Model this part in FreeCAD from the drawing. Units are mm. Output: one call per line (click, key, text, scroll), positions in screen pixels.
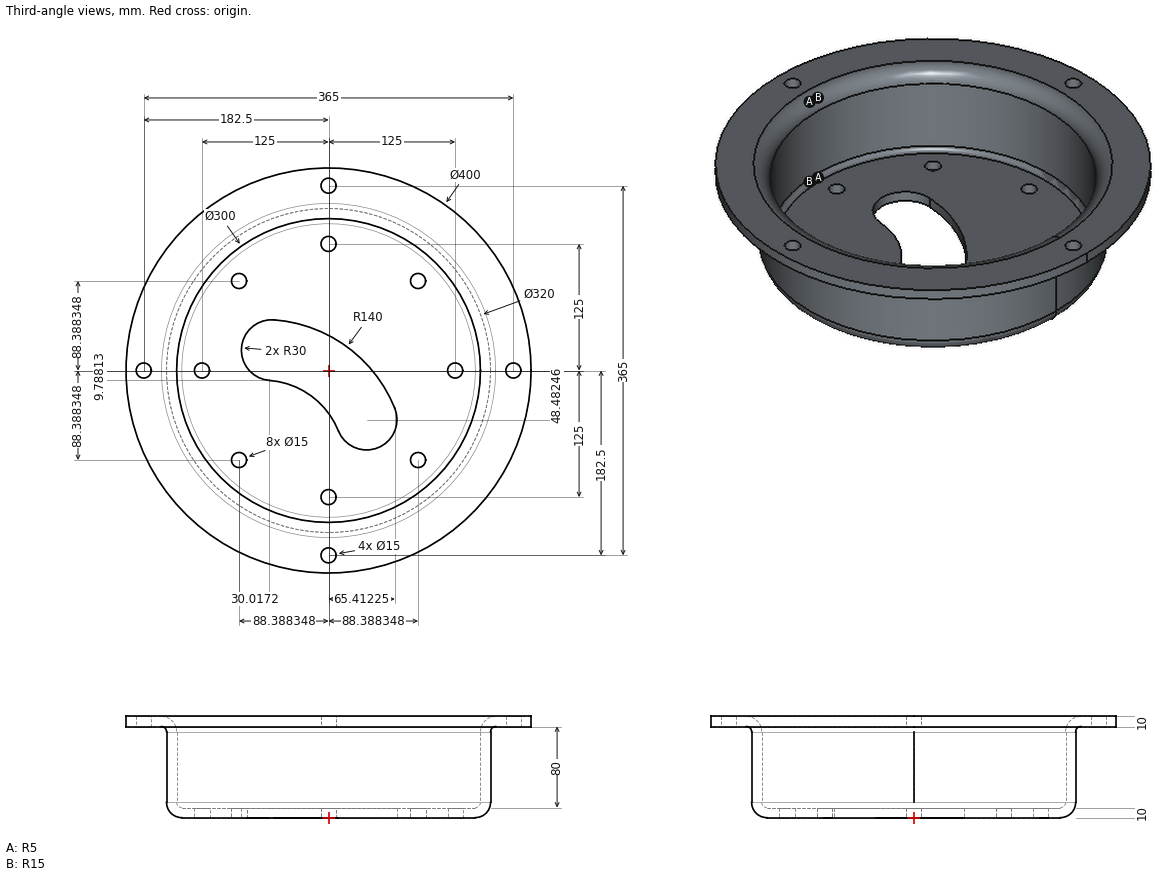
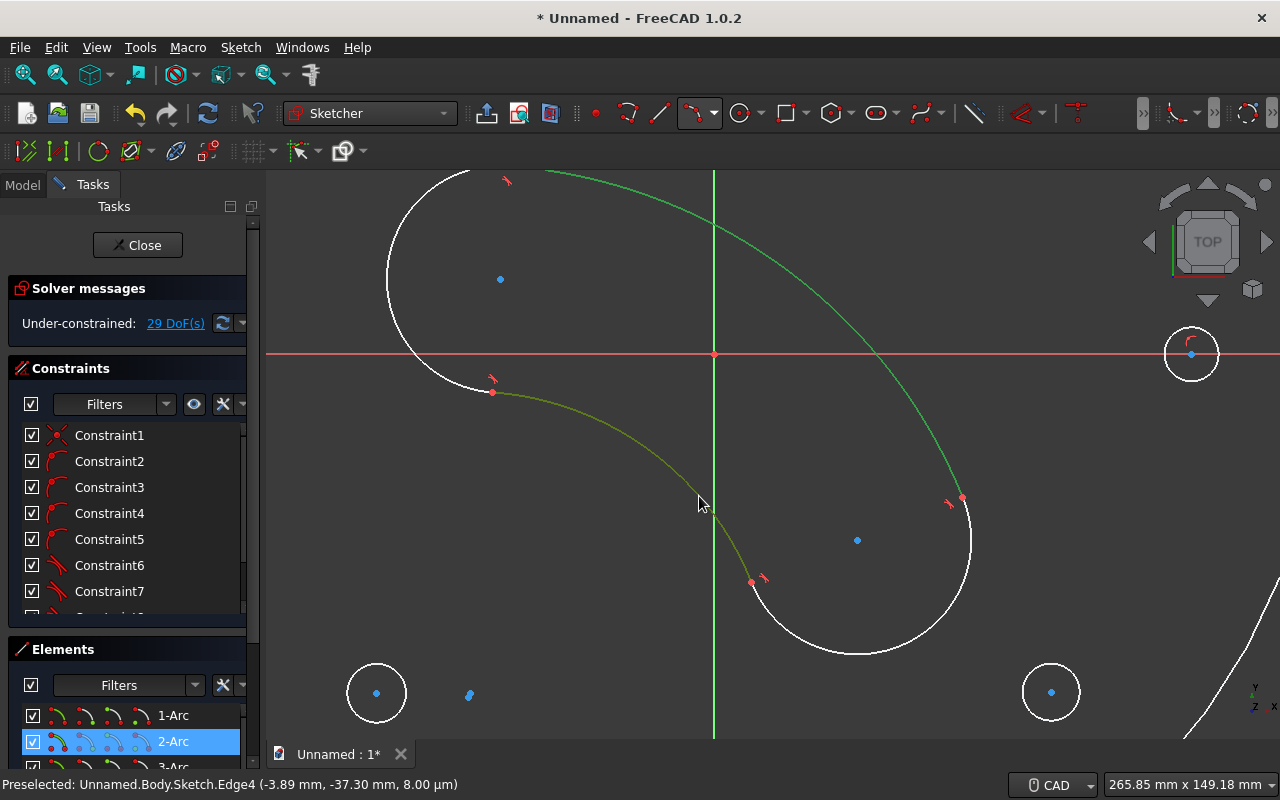
click(1076, 114)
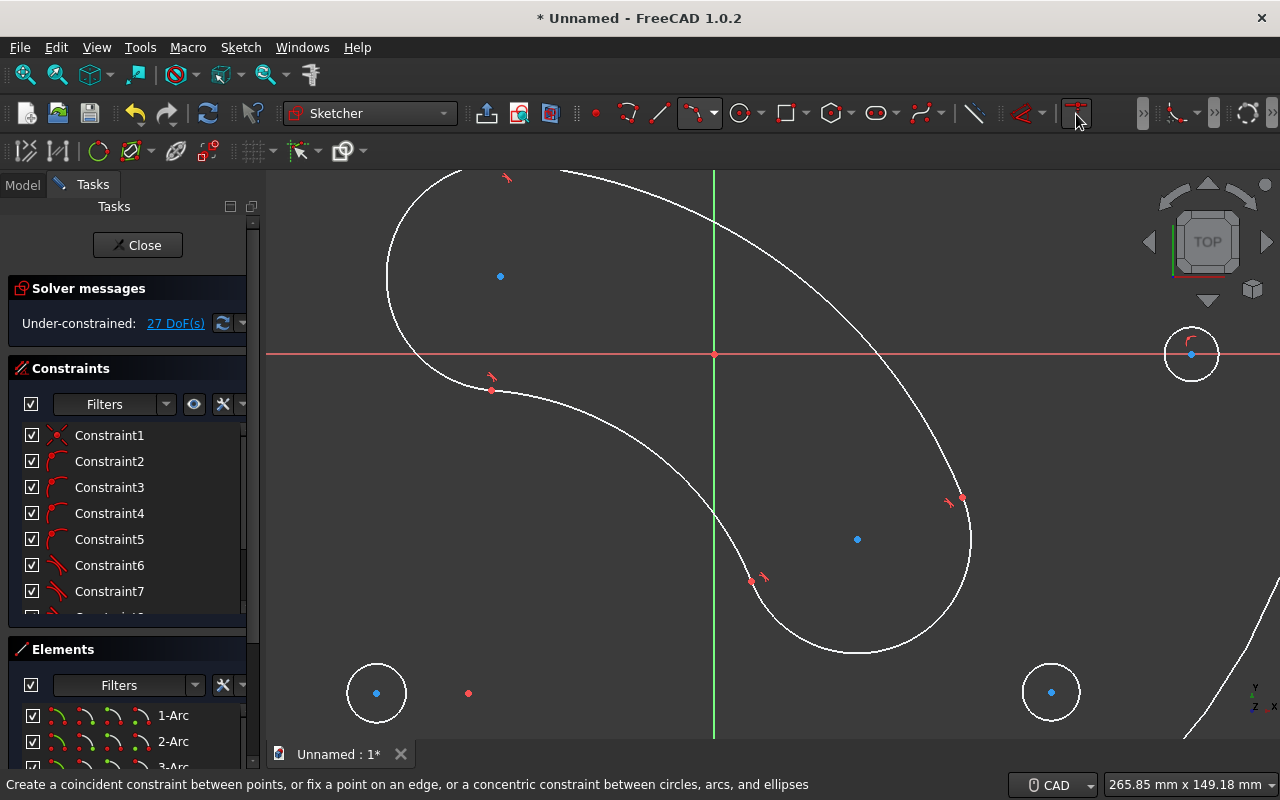
click(397, 672)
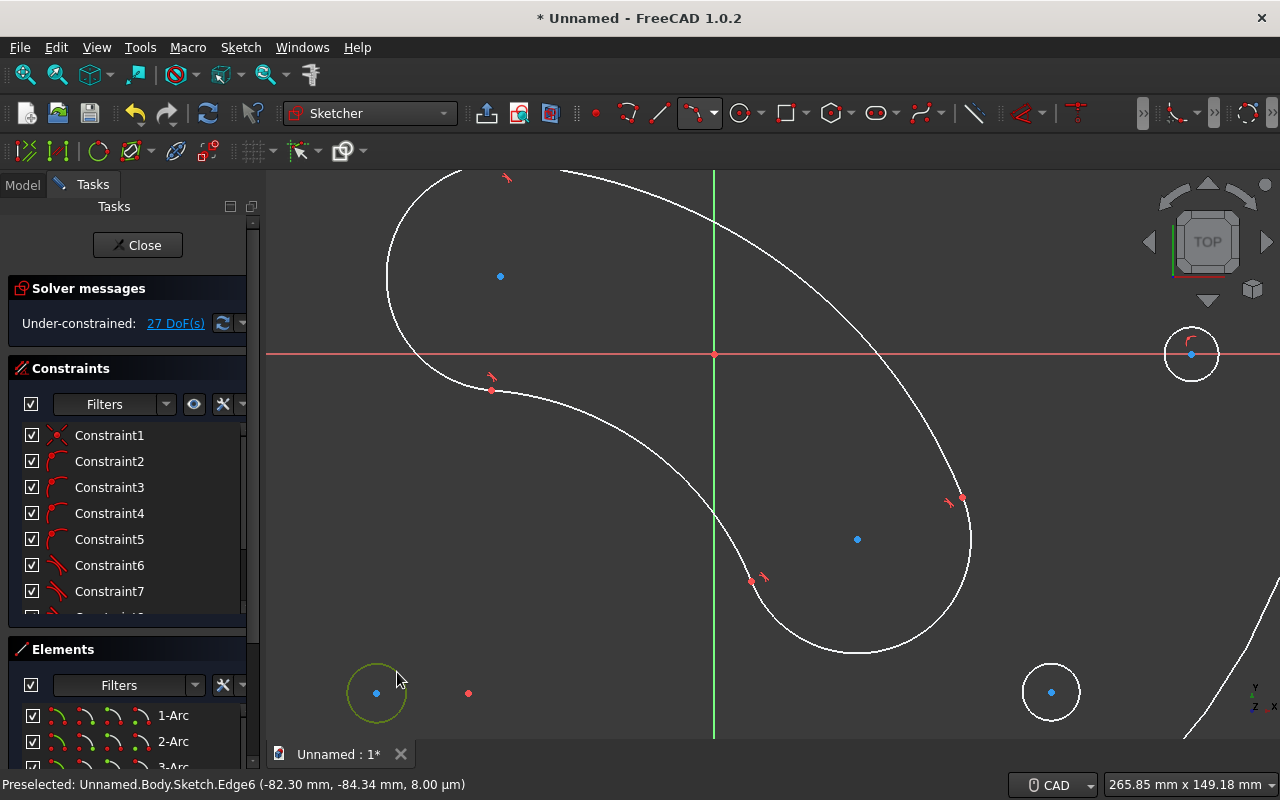
scroll(700, 498, down, 6)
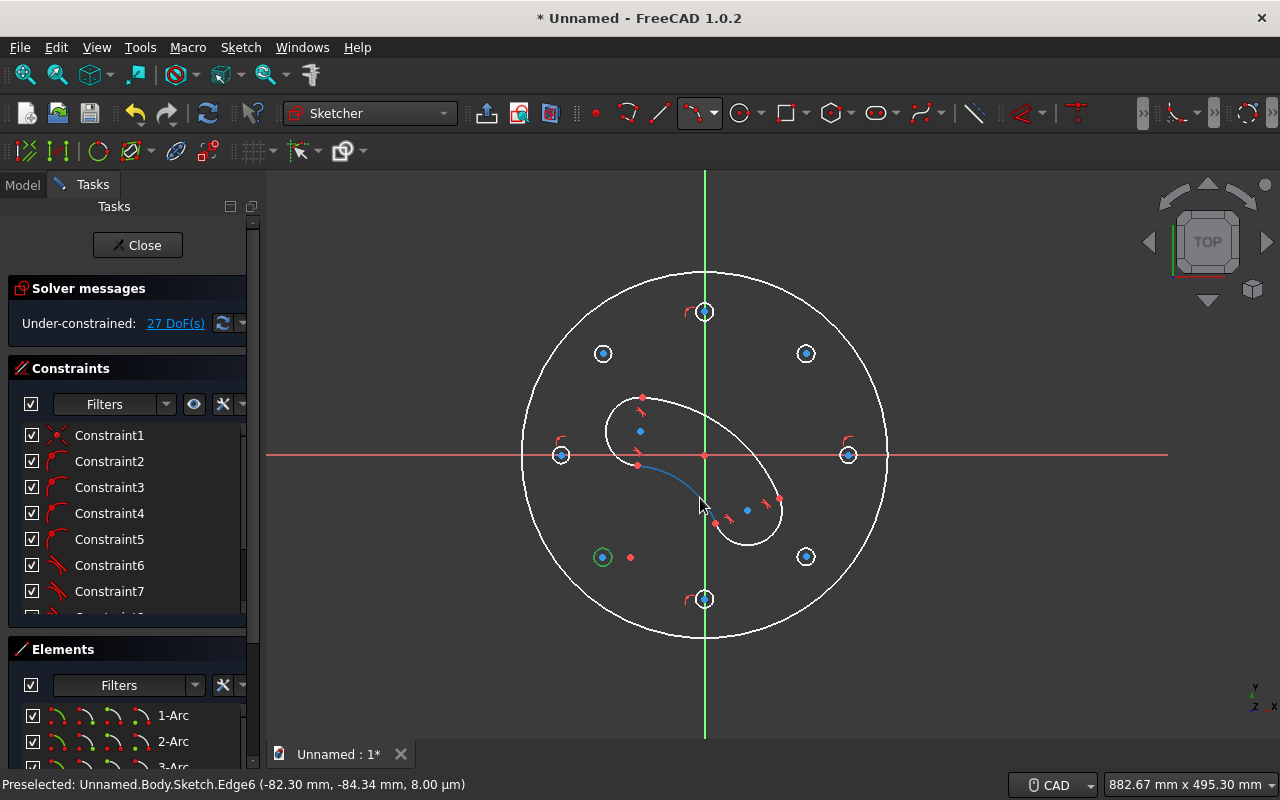
scroll(711, 593, up, 5)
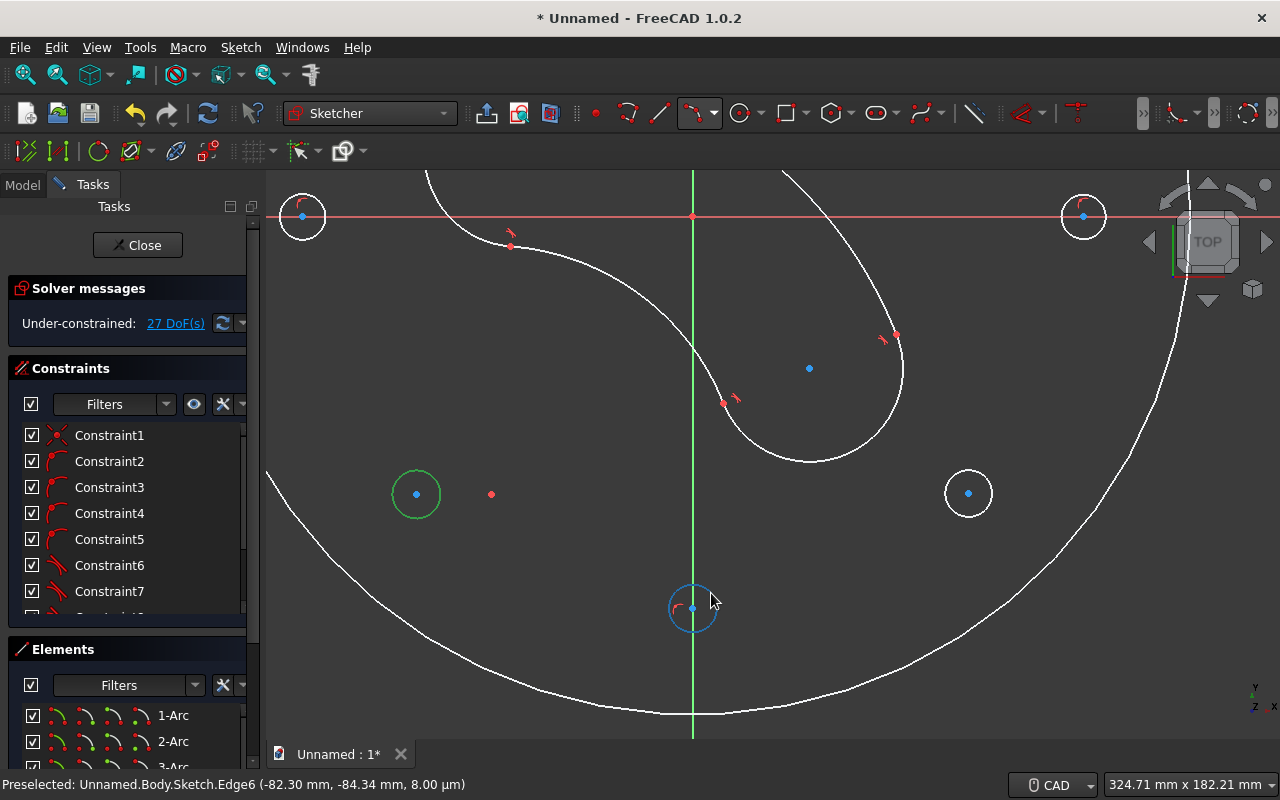
click(710, 592)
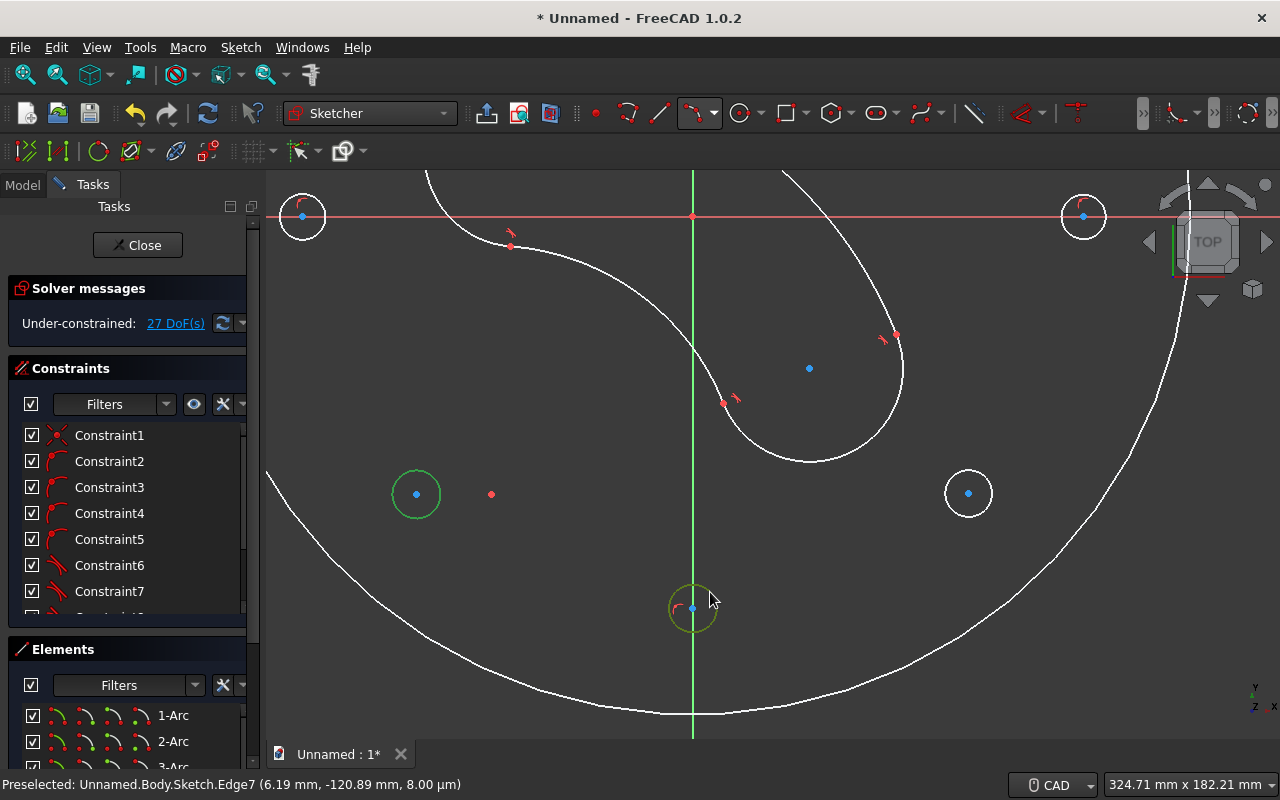
click(985, 477)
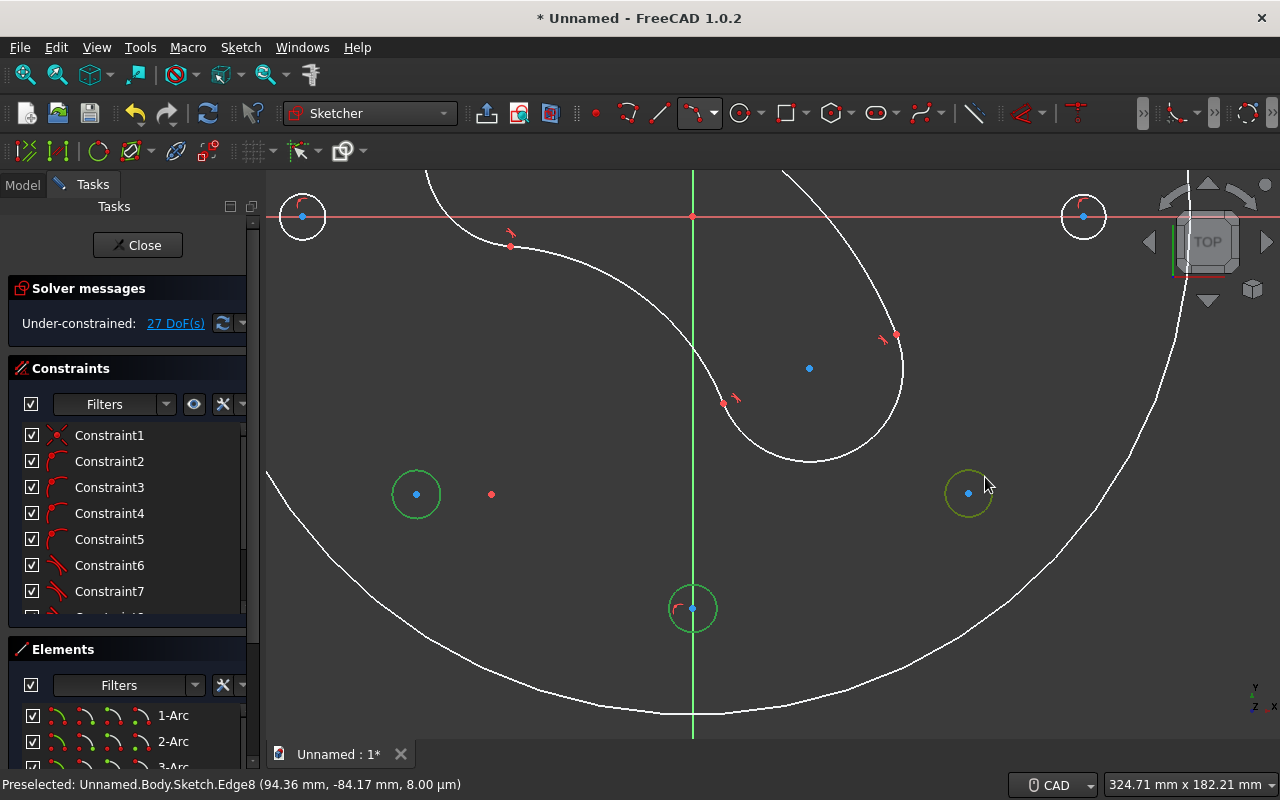
click(319, 201)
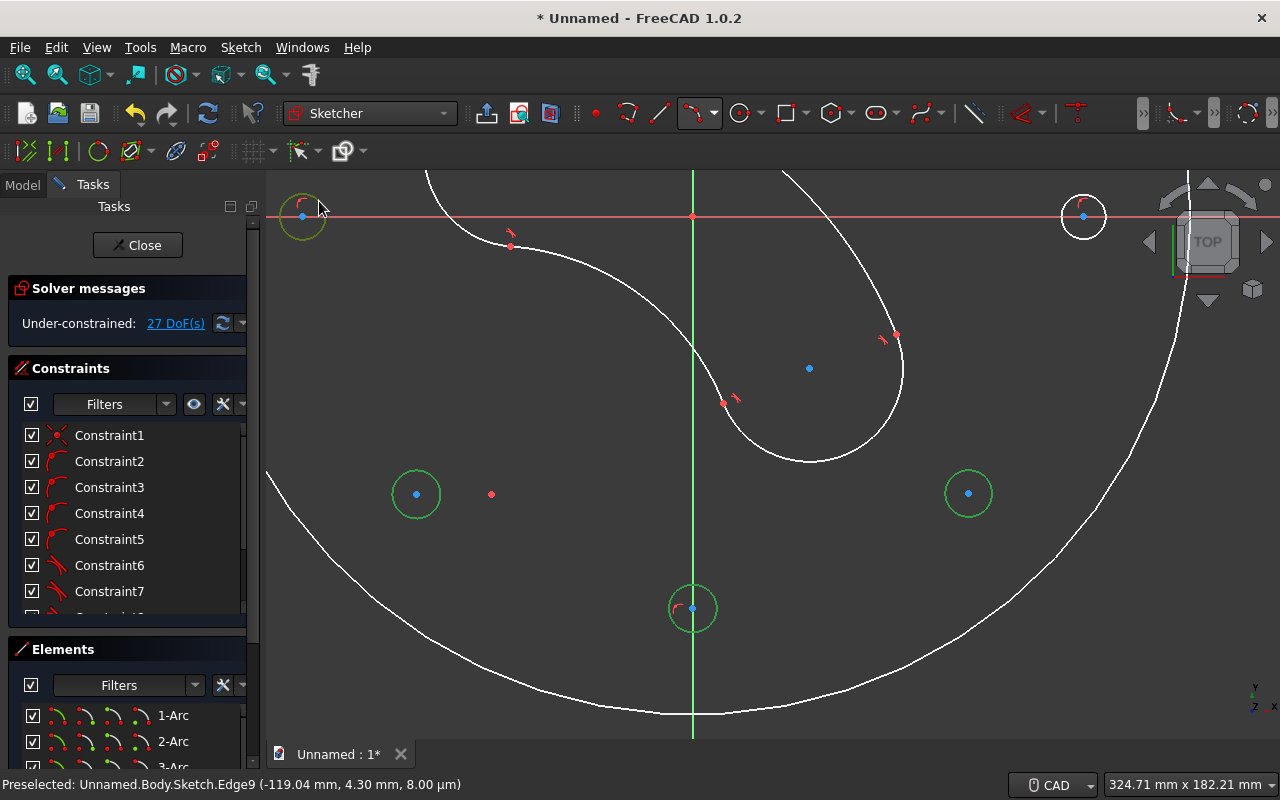
scroll(711, 593, down, 5)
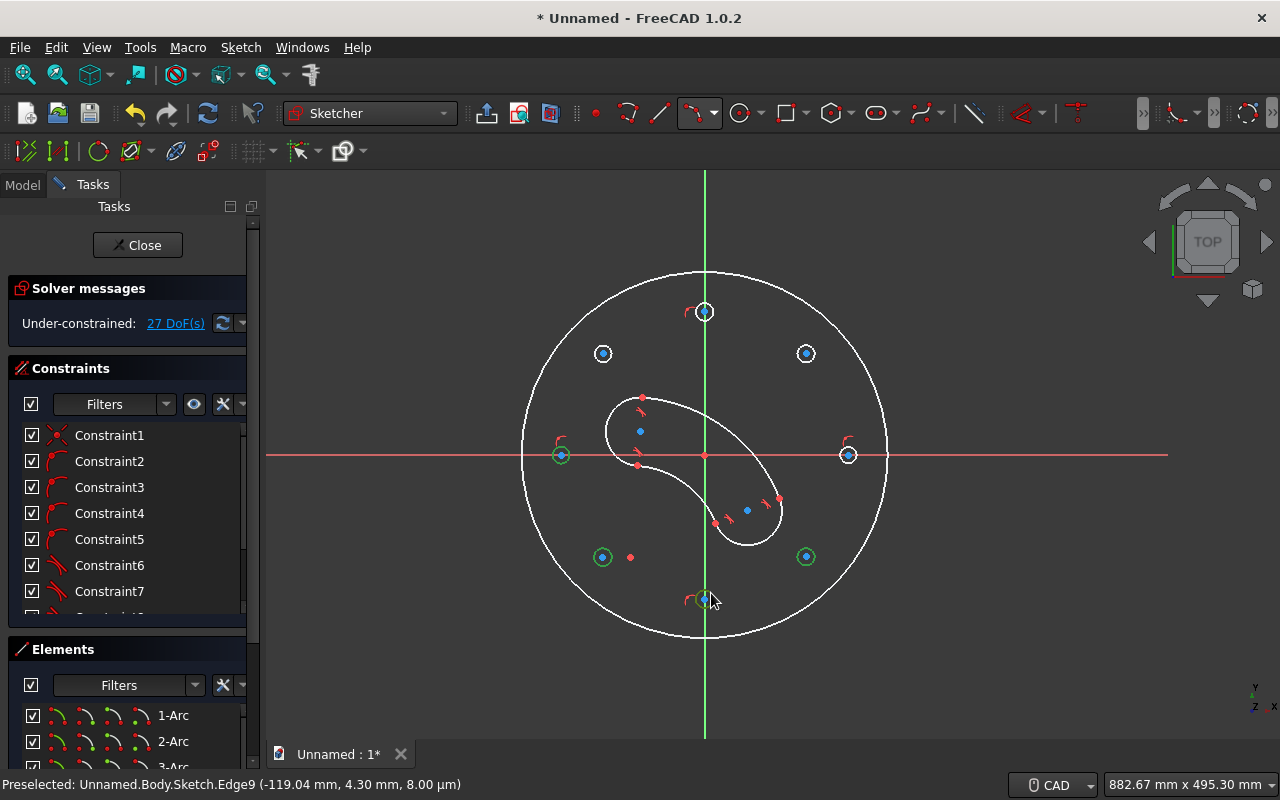
scroll(609, 348, up, 3)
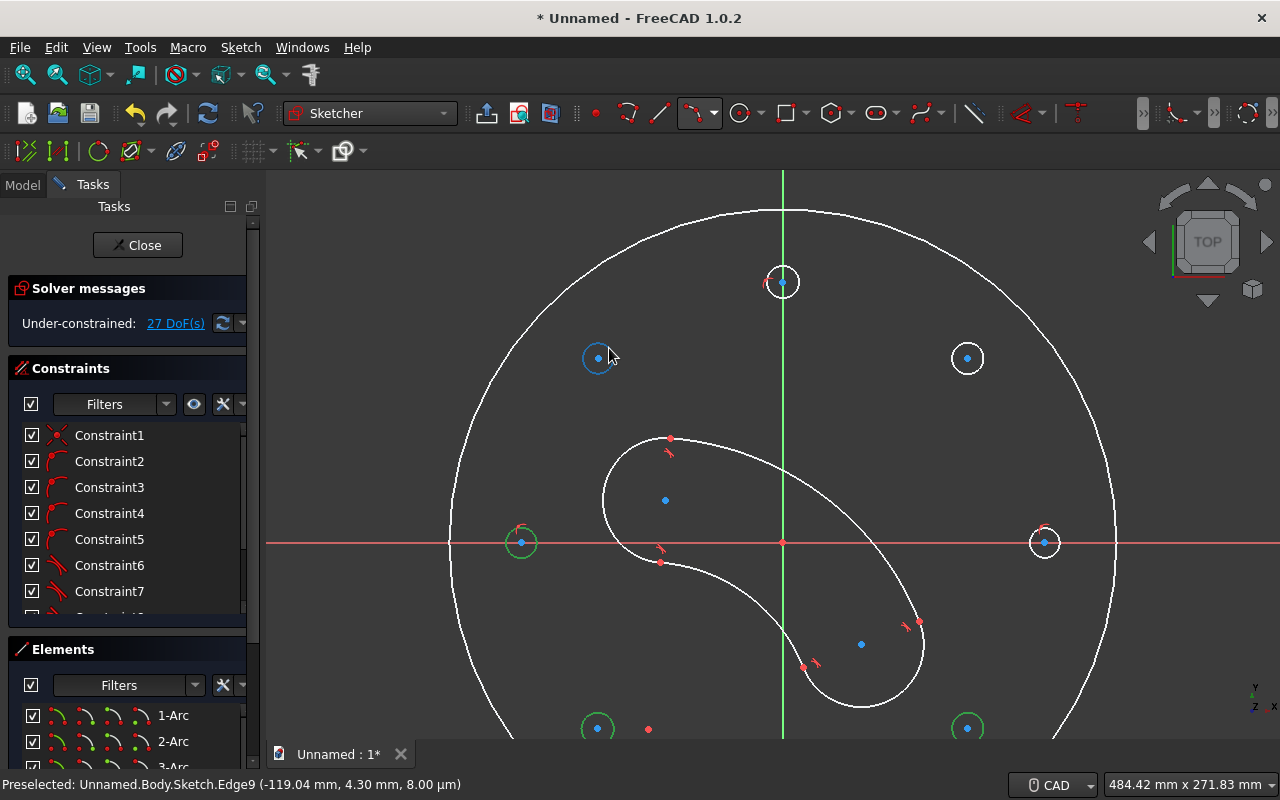
click(609, 348)